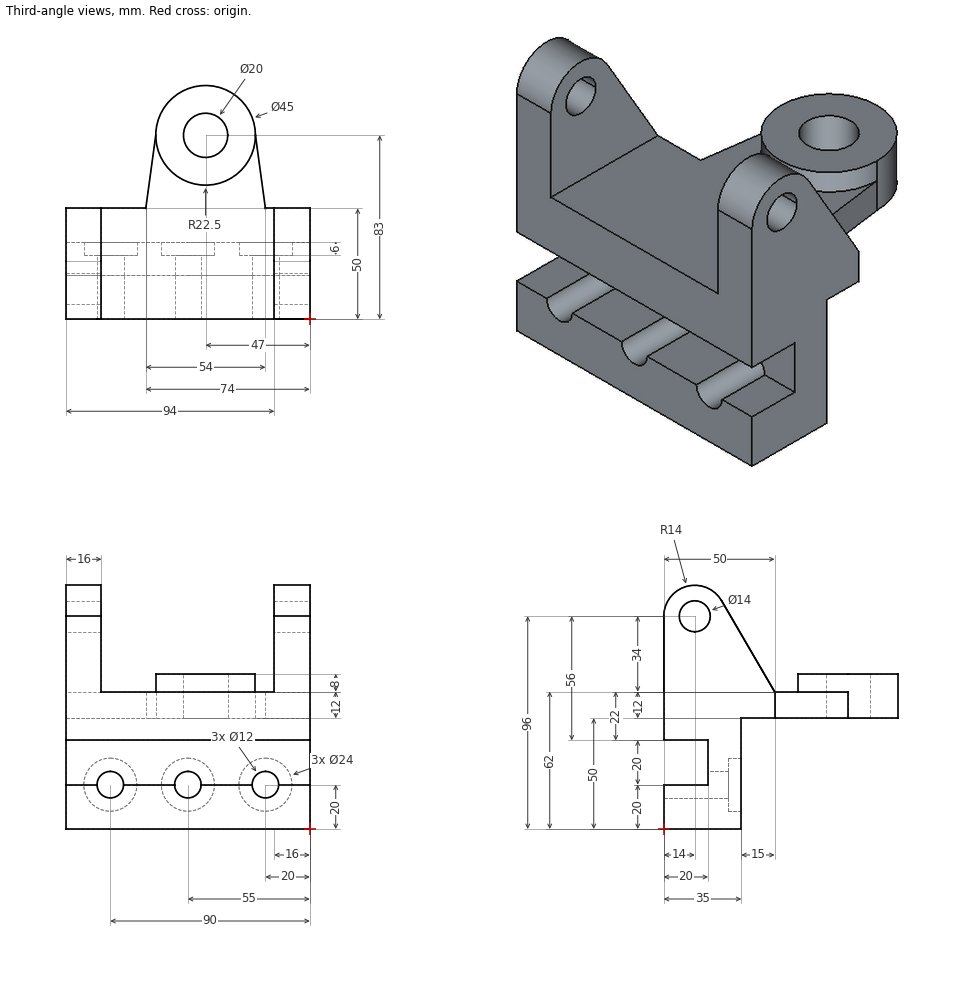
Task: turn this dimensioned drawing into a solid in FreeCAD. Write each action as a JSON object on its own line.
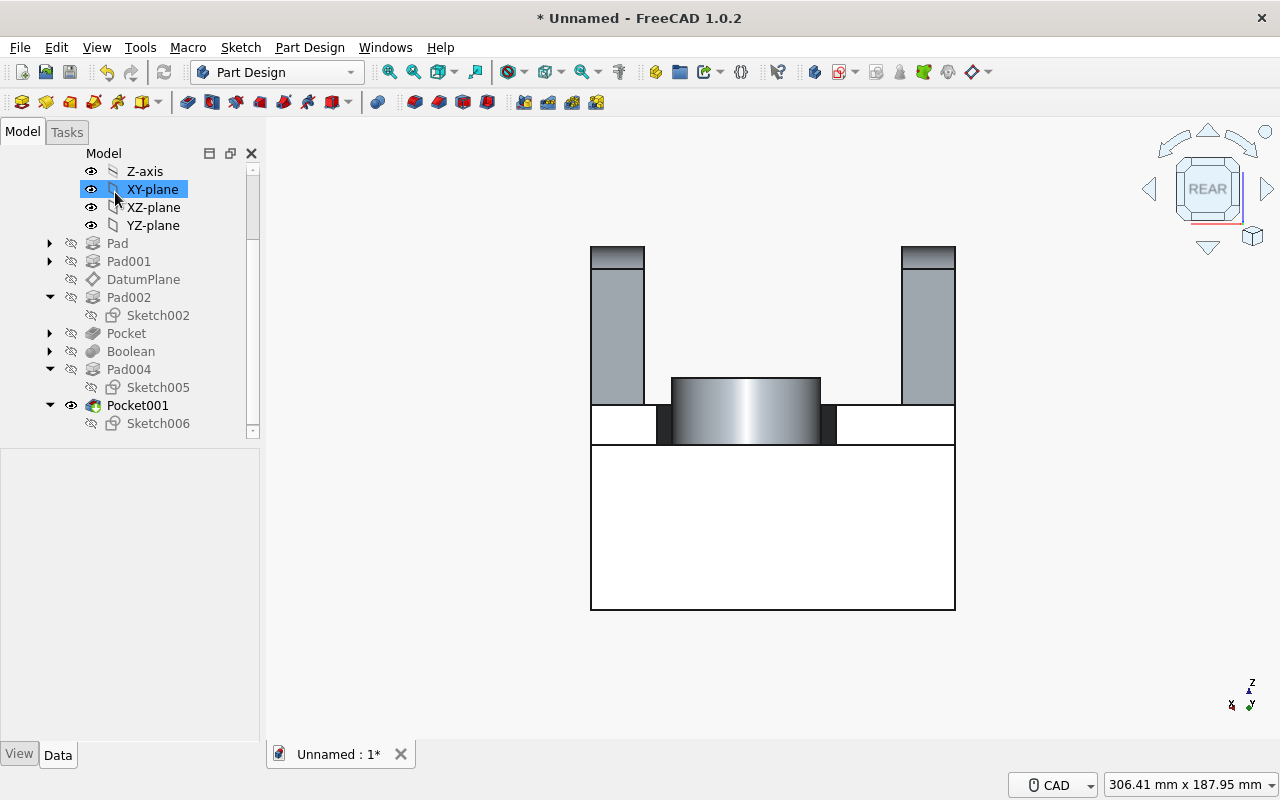
{"action": "left_click", "coordinate": [773, 526]}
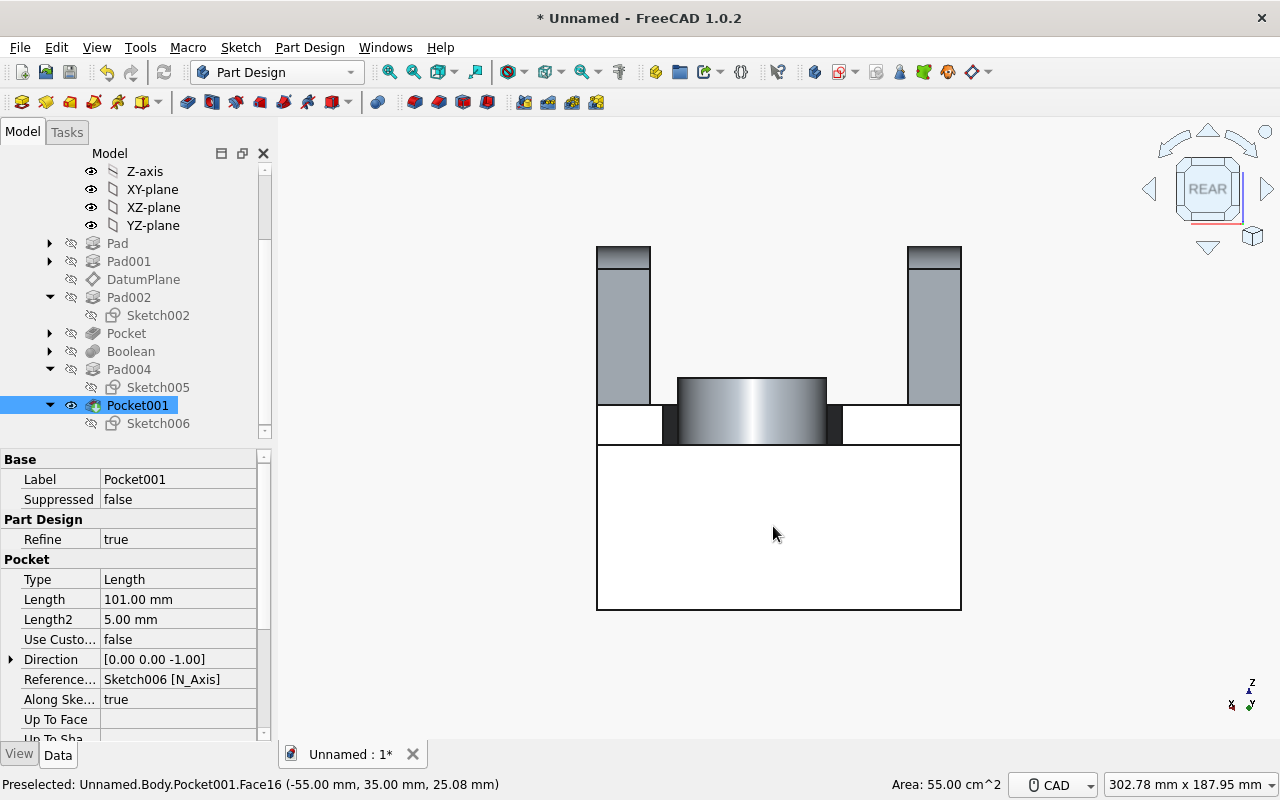
{"action": "left_click", "coordinate": [840, 72]}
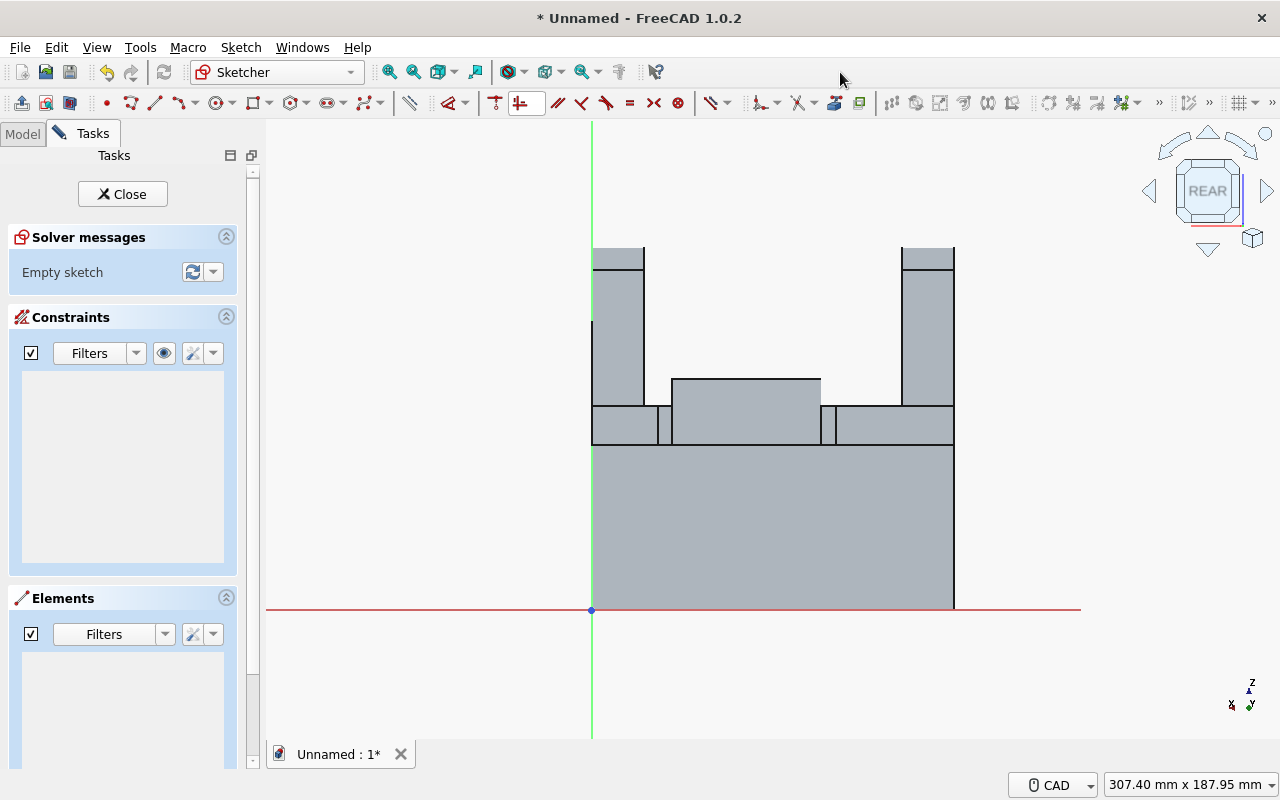
{"action": "left_click", "coordinate": [70, 104]}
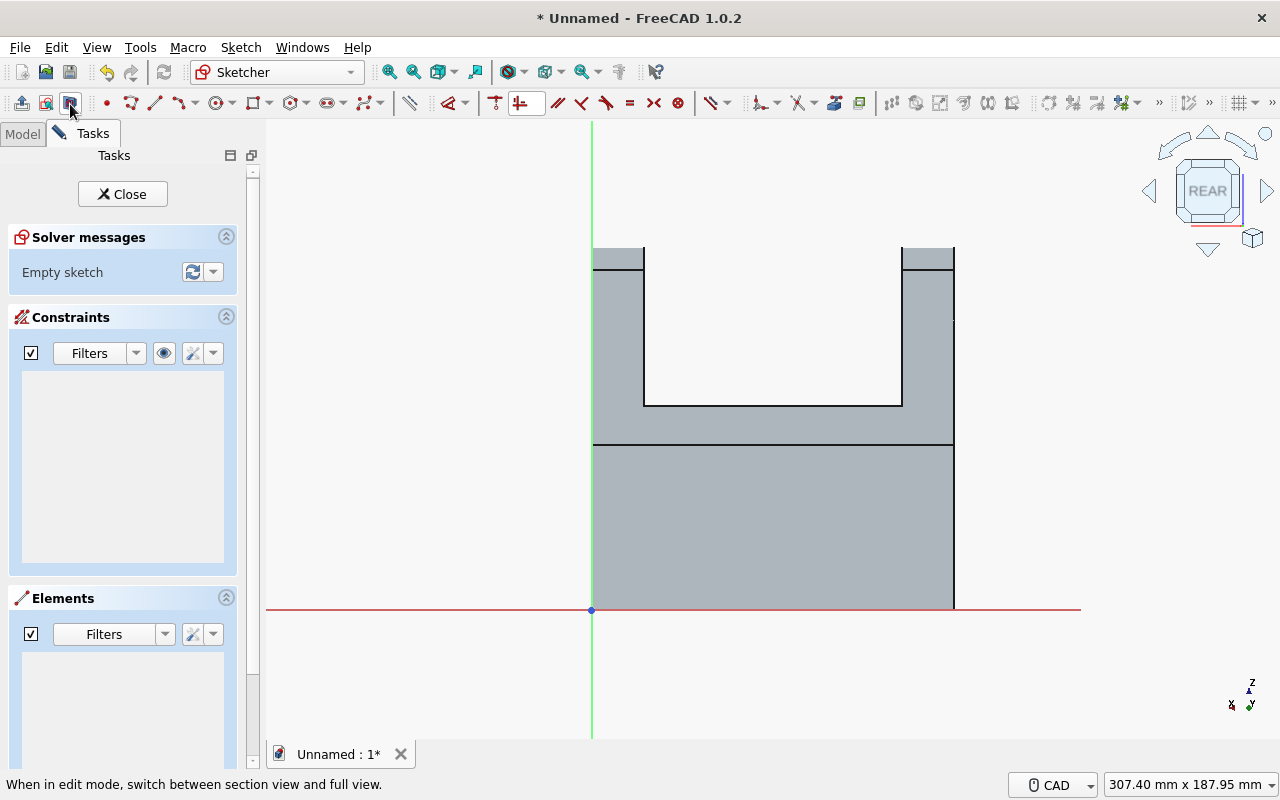
{"action": "scroll", "coordinate": [827, 711], "scroll_direction": "up", "scroll_amount": 3}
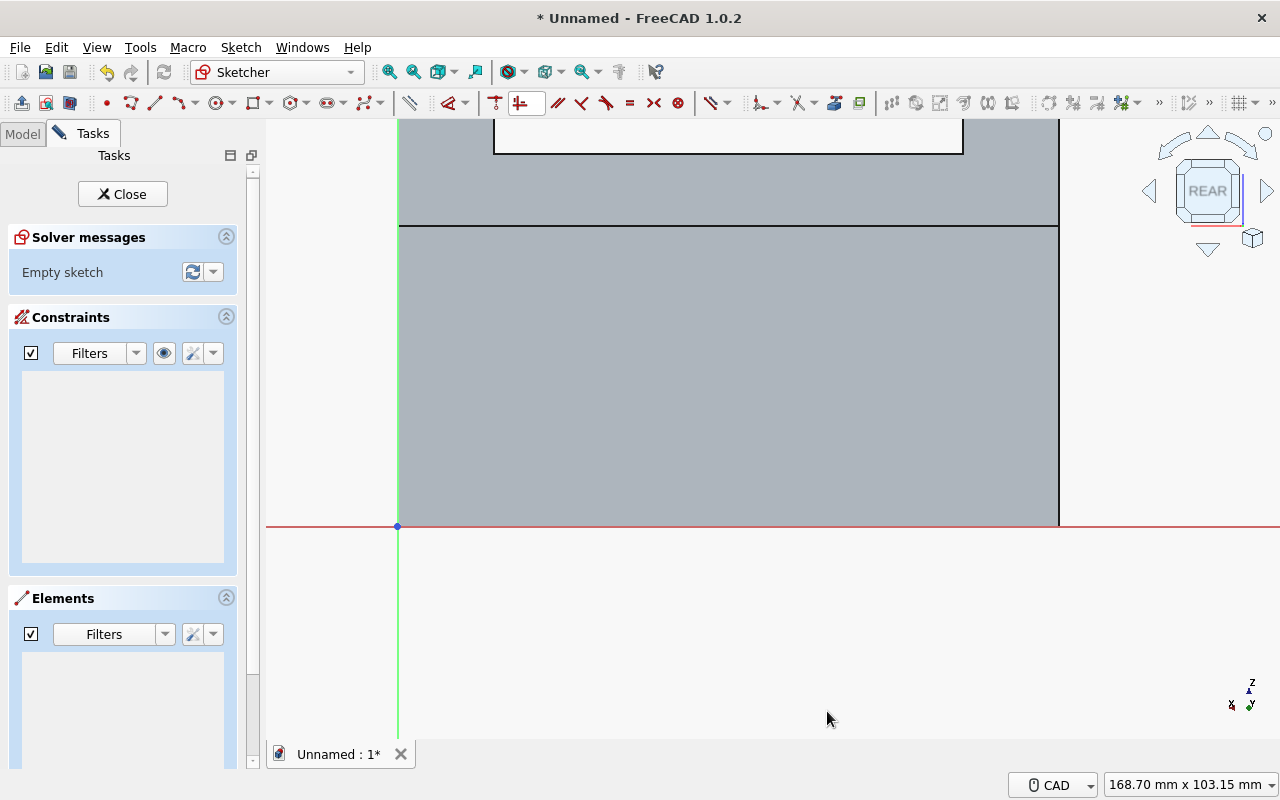
{"action": "left_click", "coordinate": [216, 104]}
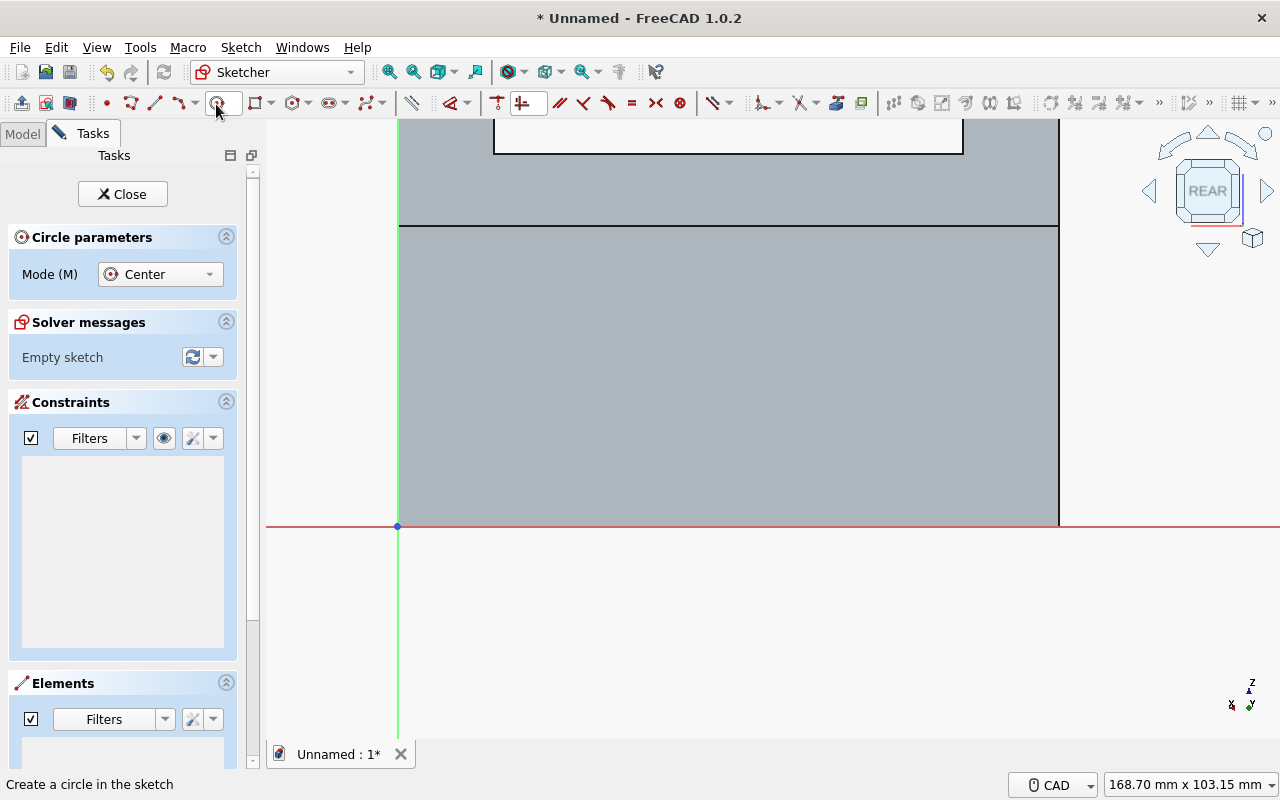
{"action": "left_click", "coordinate": [518, 407]}
{"action": "mouse_move", "coordinate": [569, 356]}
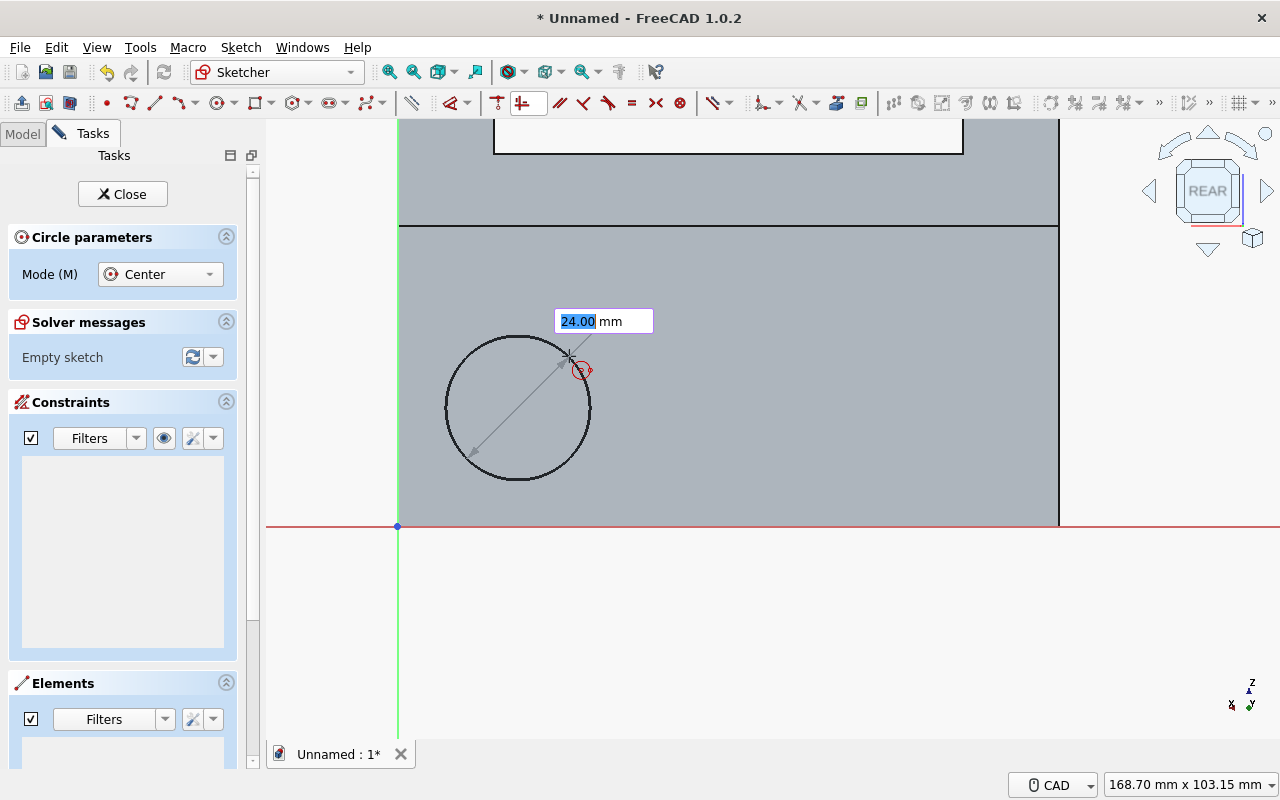
{"action": "type", "text": "24"}
{"action": "key", "text": "Return"}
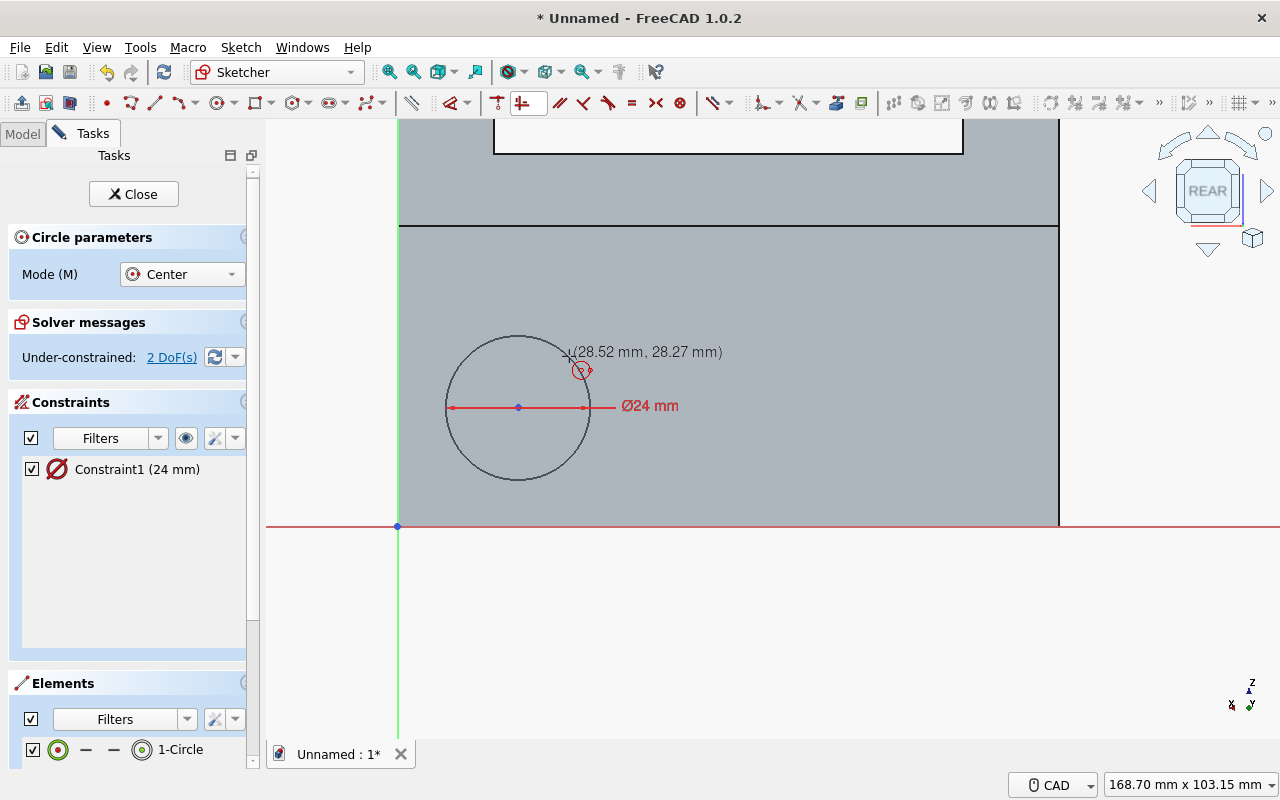
{"action": "left_click", "coordinate": [728, 407]}
{"action": "mouse_move", "coordinate": [779, 356]}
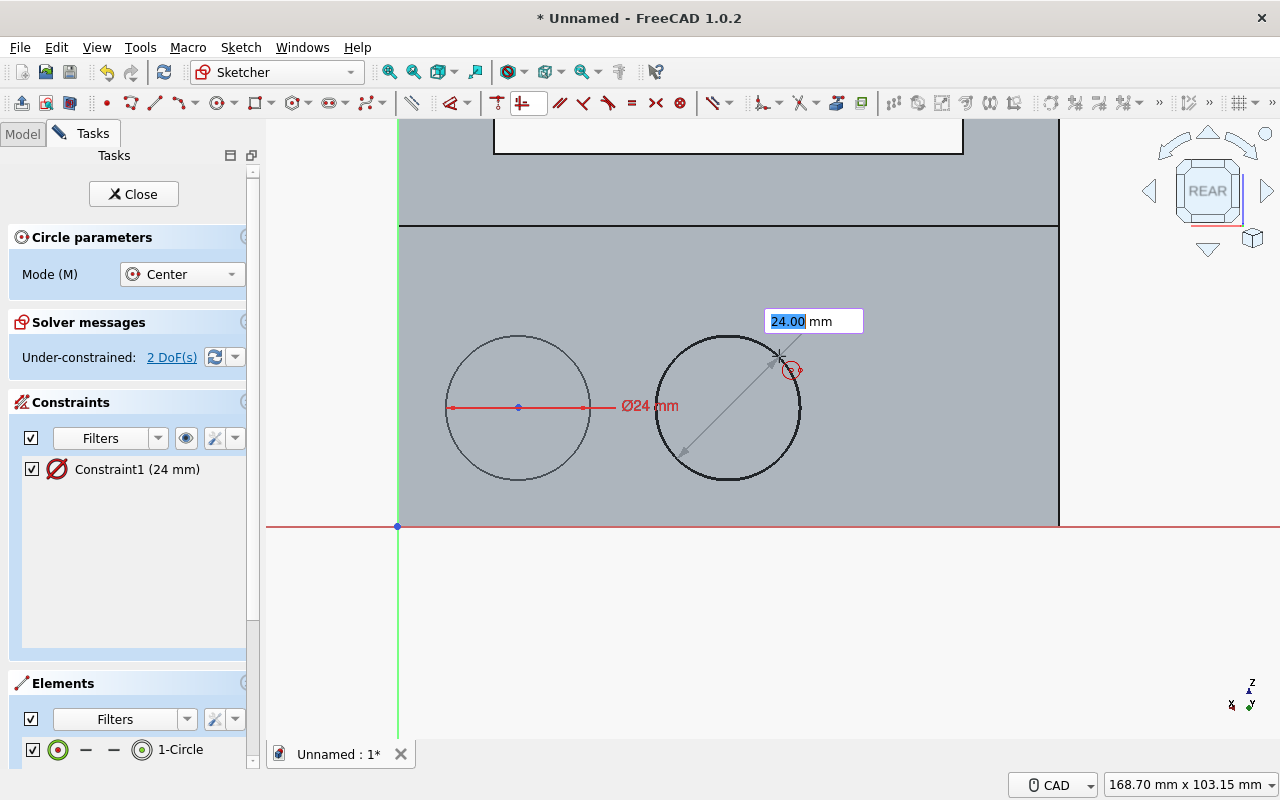
{"action": "type", "text": "24"}
{"action": "key", "text": "Return"}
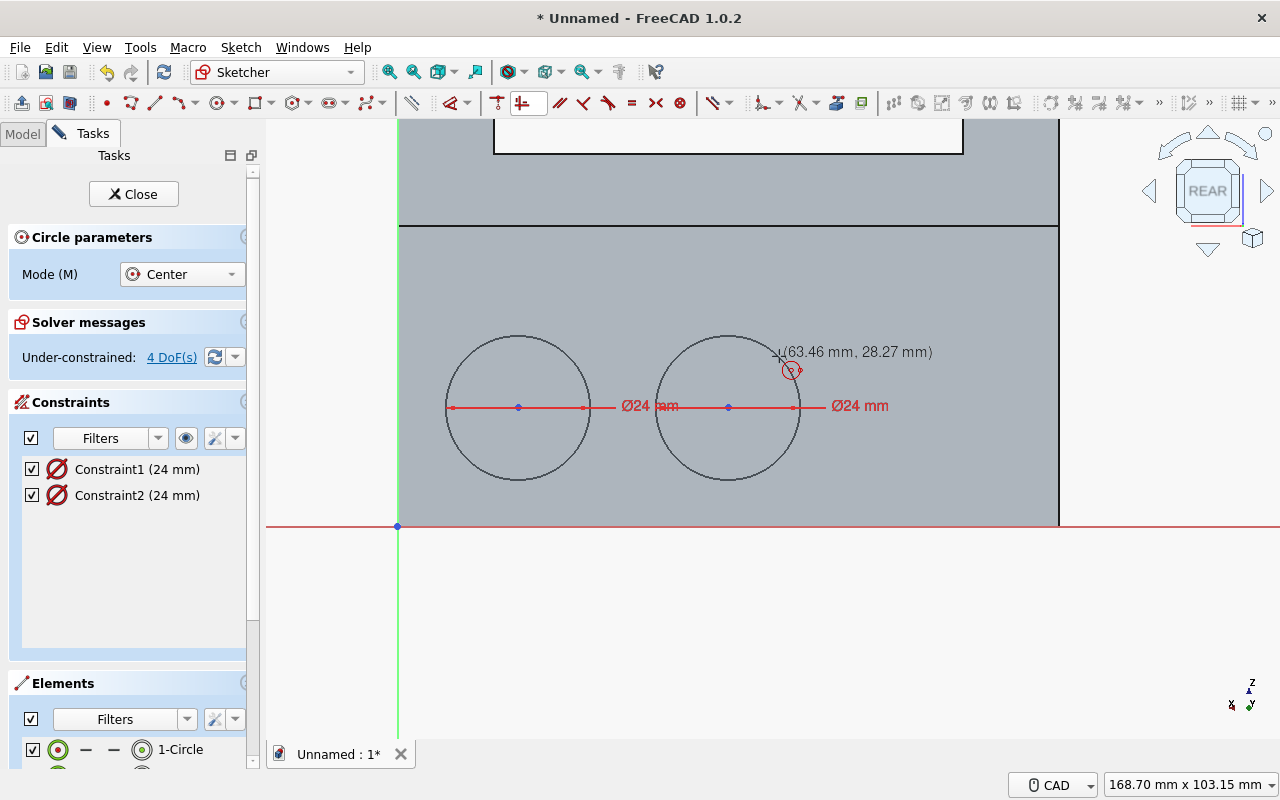
{"action": "left_click", "coordinate": [939, 407]}
{"action": "mouse_move", "coordinate": [990, 356]}